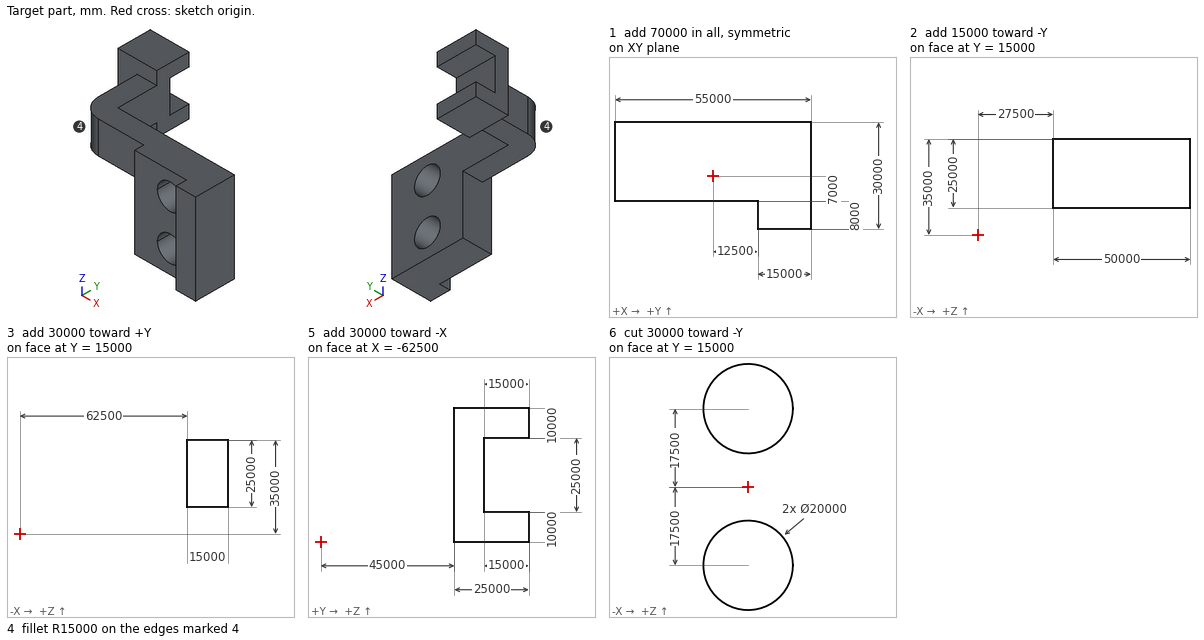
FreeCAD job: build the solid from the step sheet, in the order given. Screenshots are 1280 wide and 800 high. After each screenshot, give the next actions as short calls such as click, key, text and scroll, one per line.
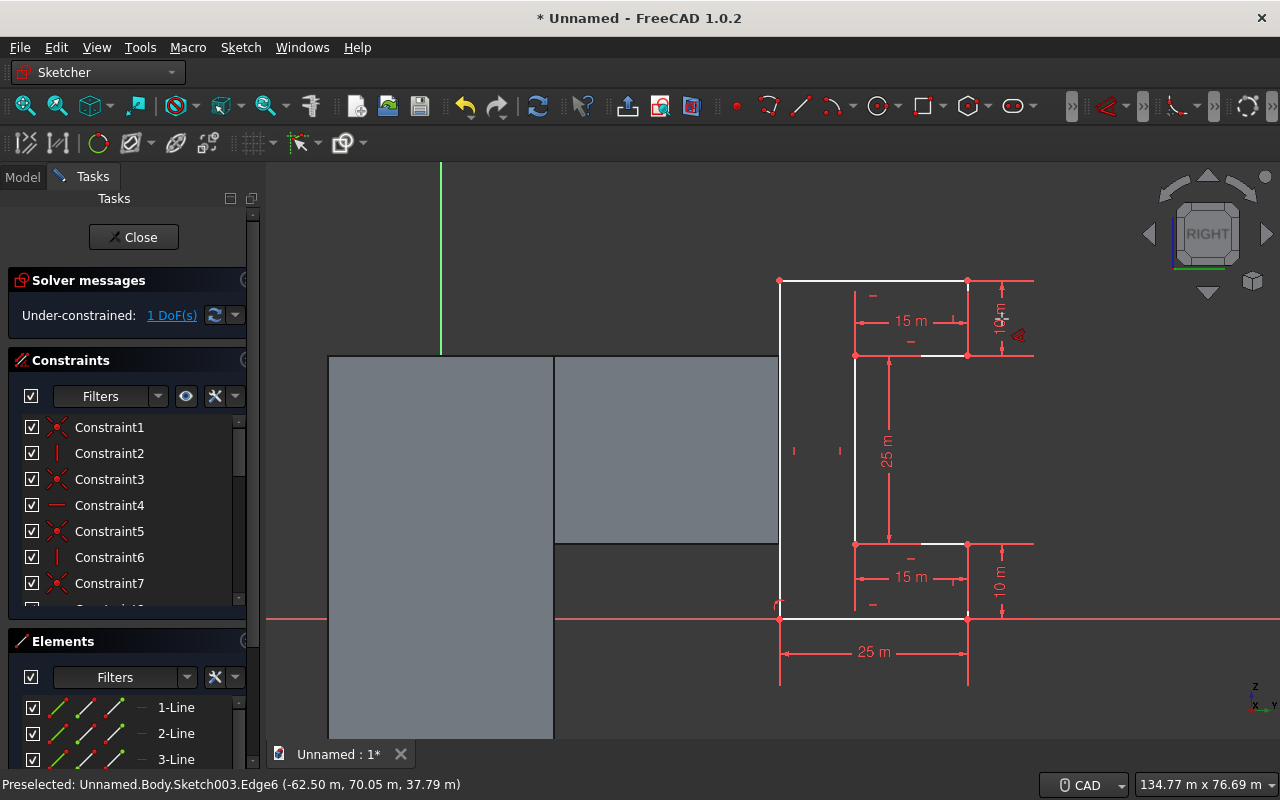
click(780, 619)
click(610, 653)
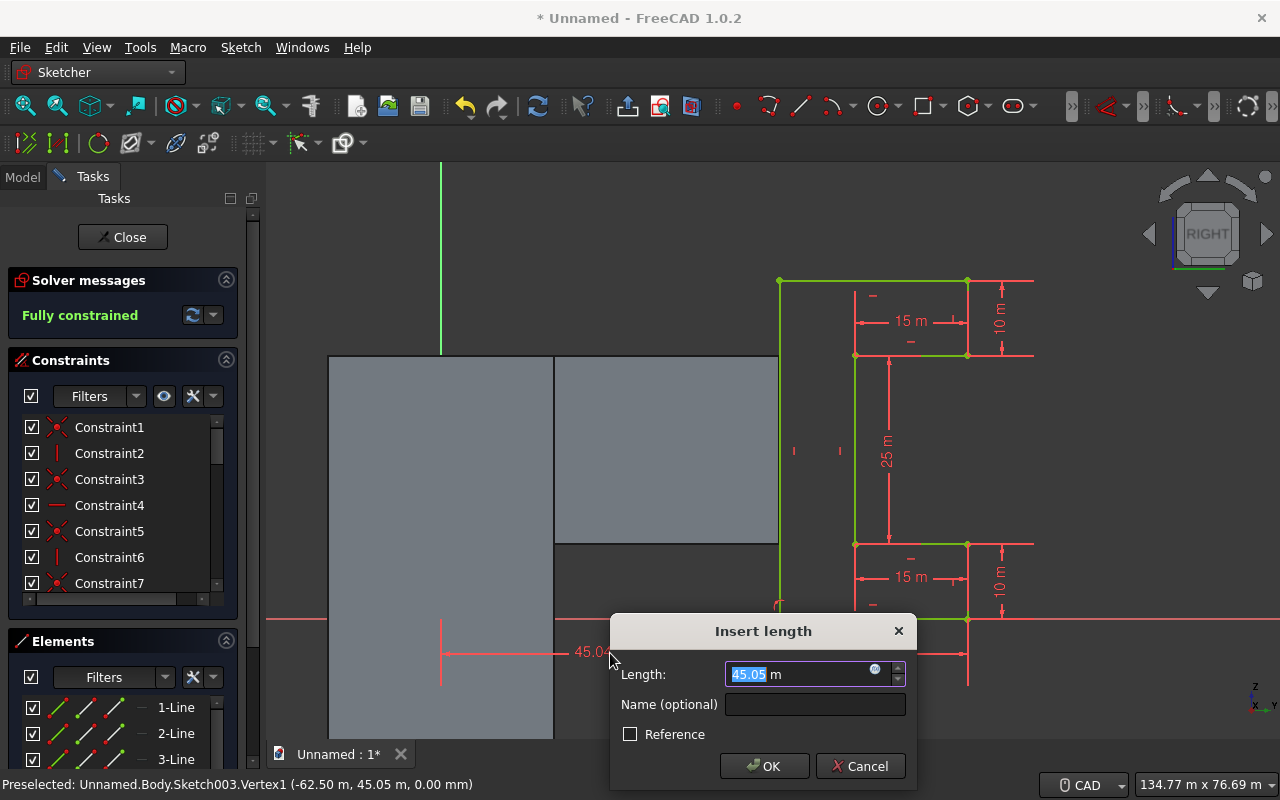
key(ctrl+a)
text(45000 mm)
key(Return)
key(Escape)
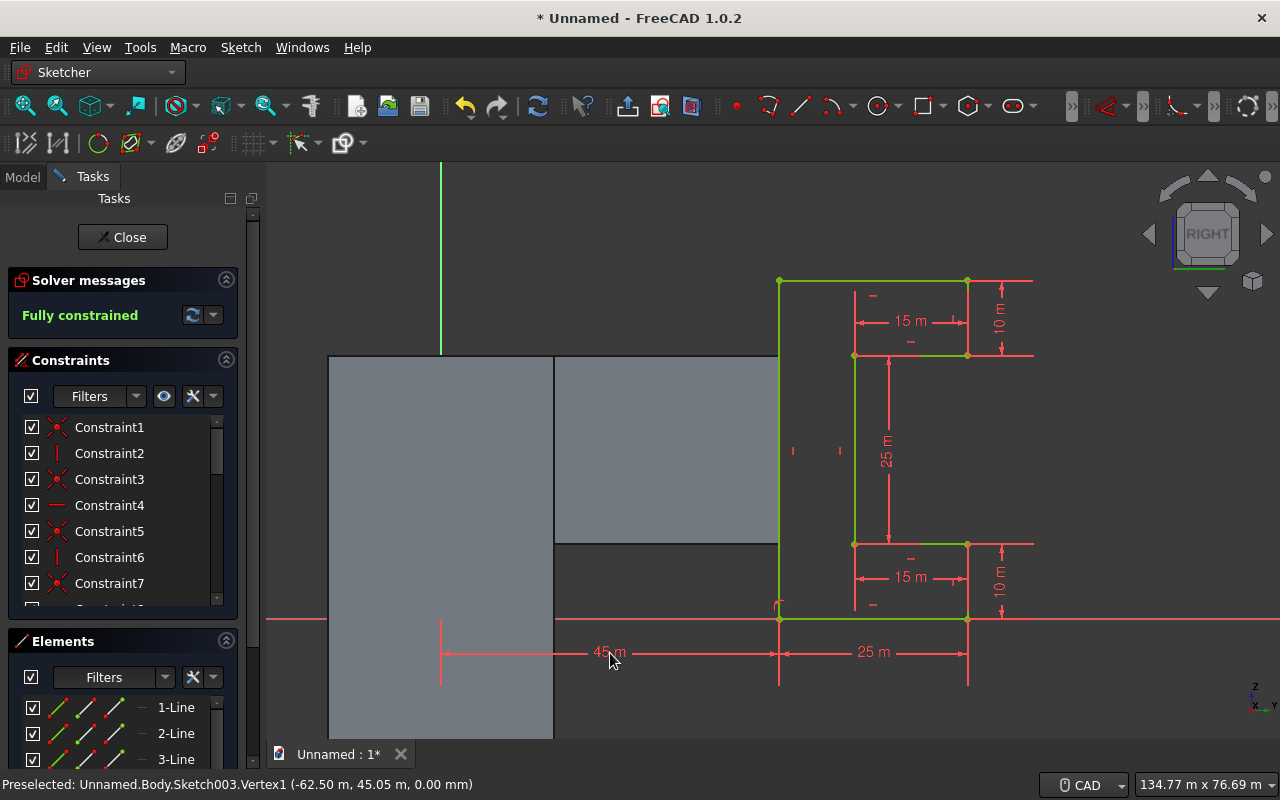
click(123, 237)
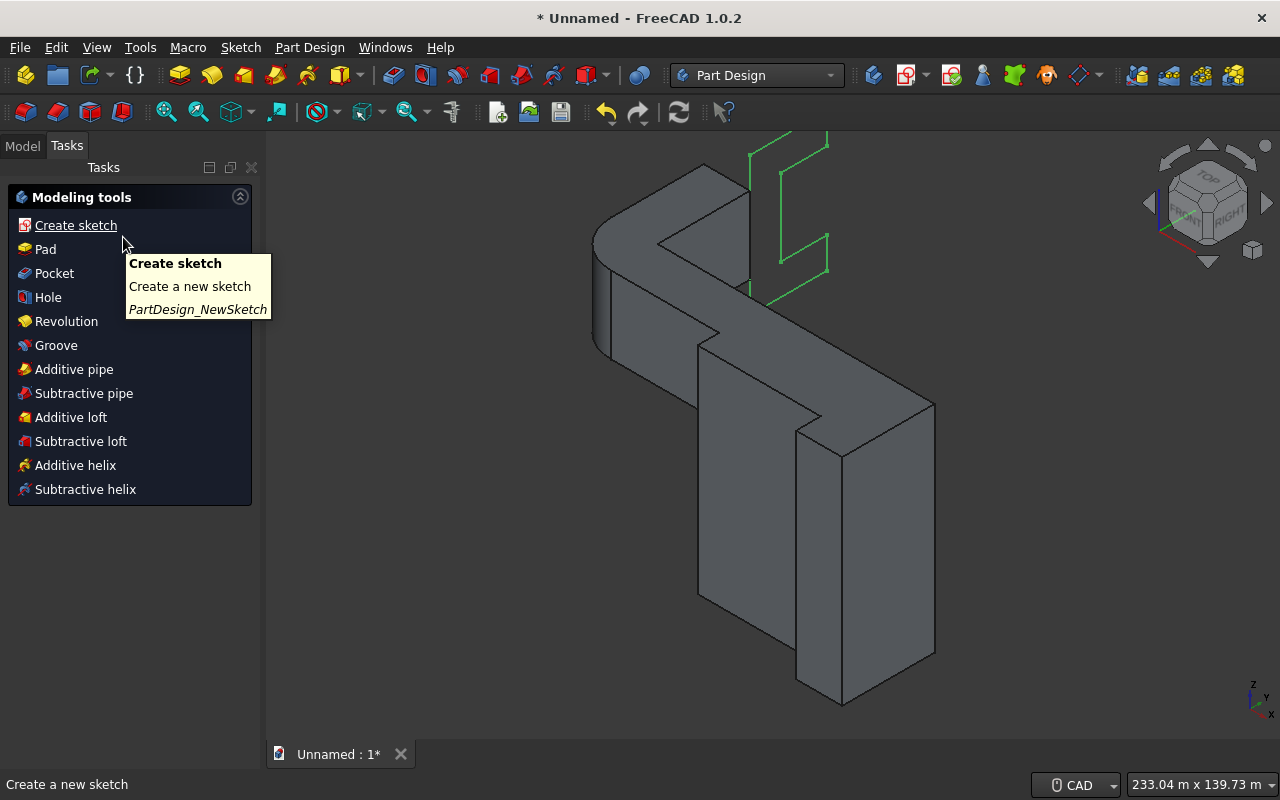
click(180, 76)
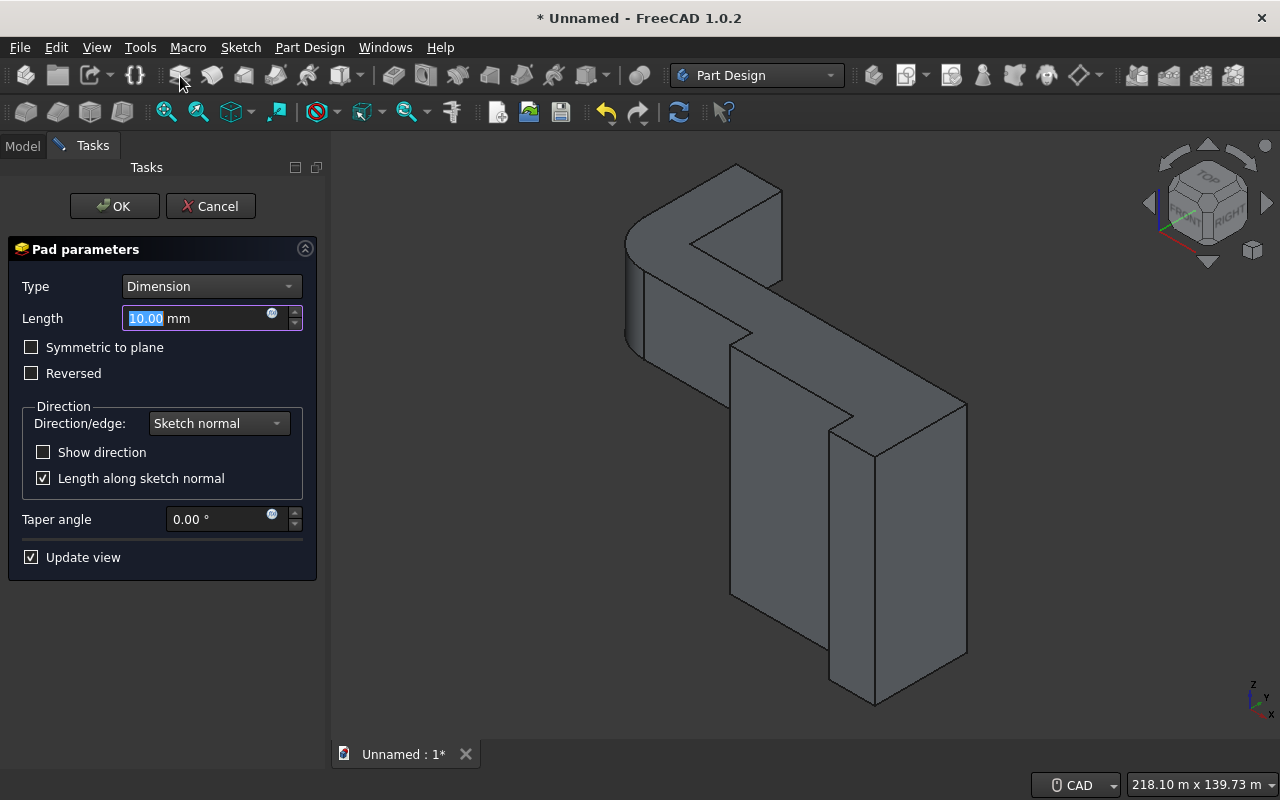
text(30000)
key(Tab)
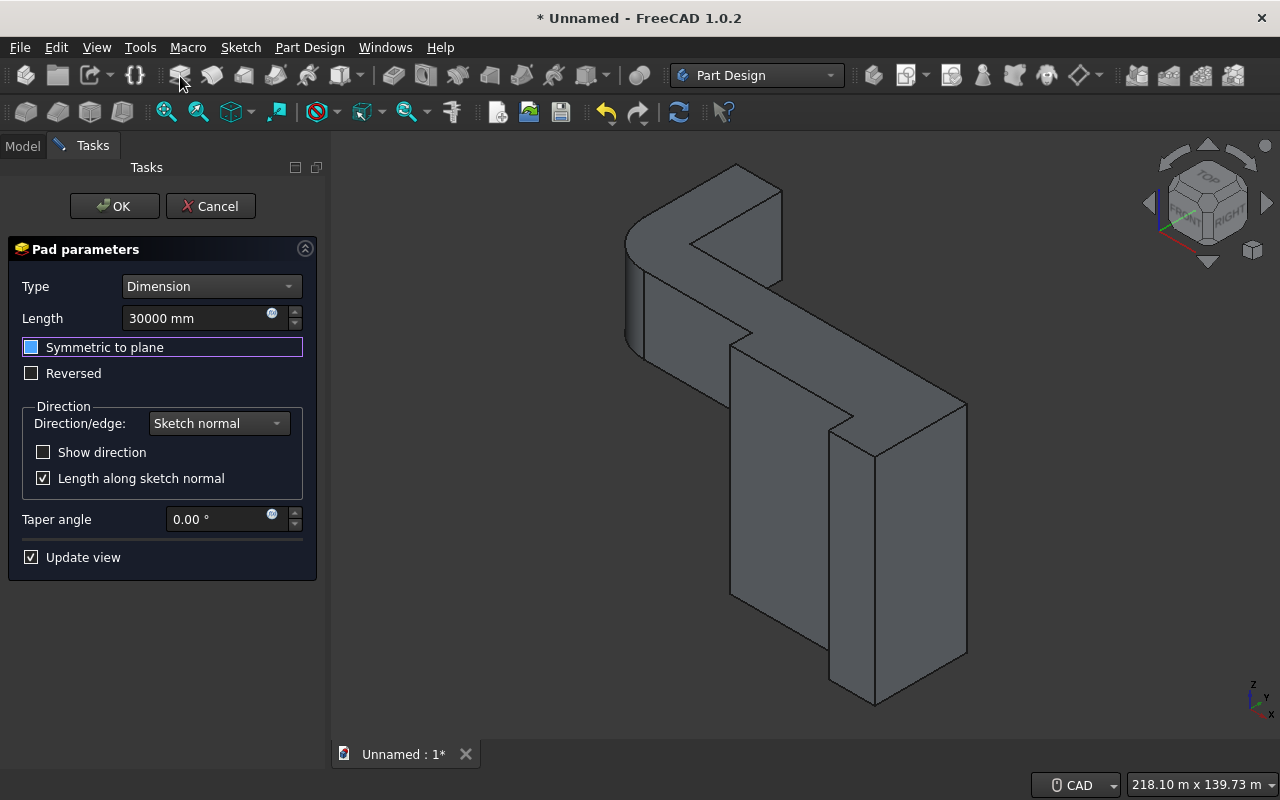
click(30, 373)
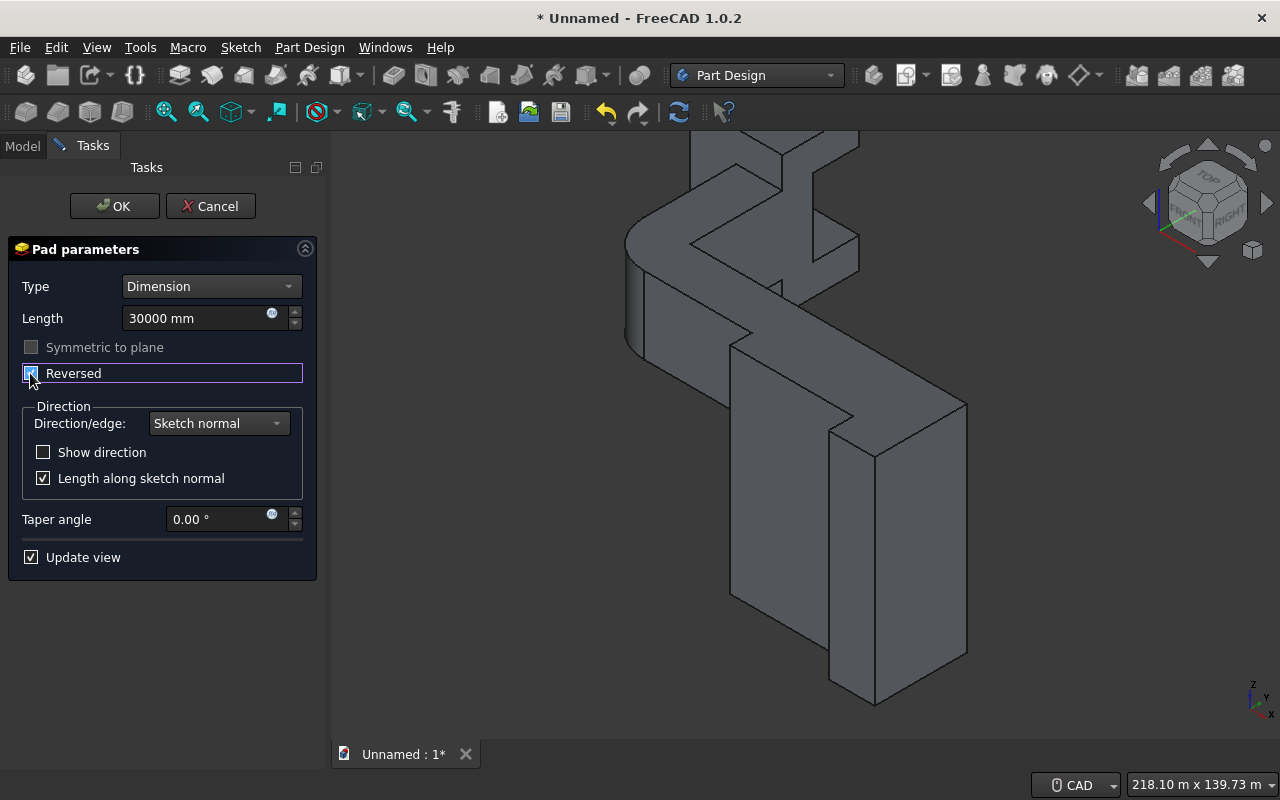
click(115, 206)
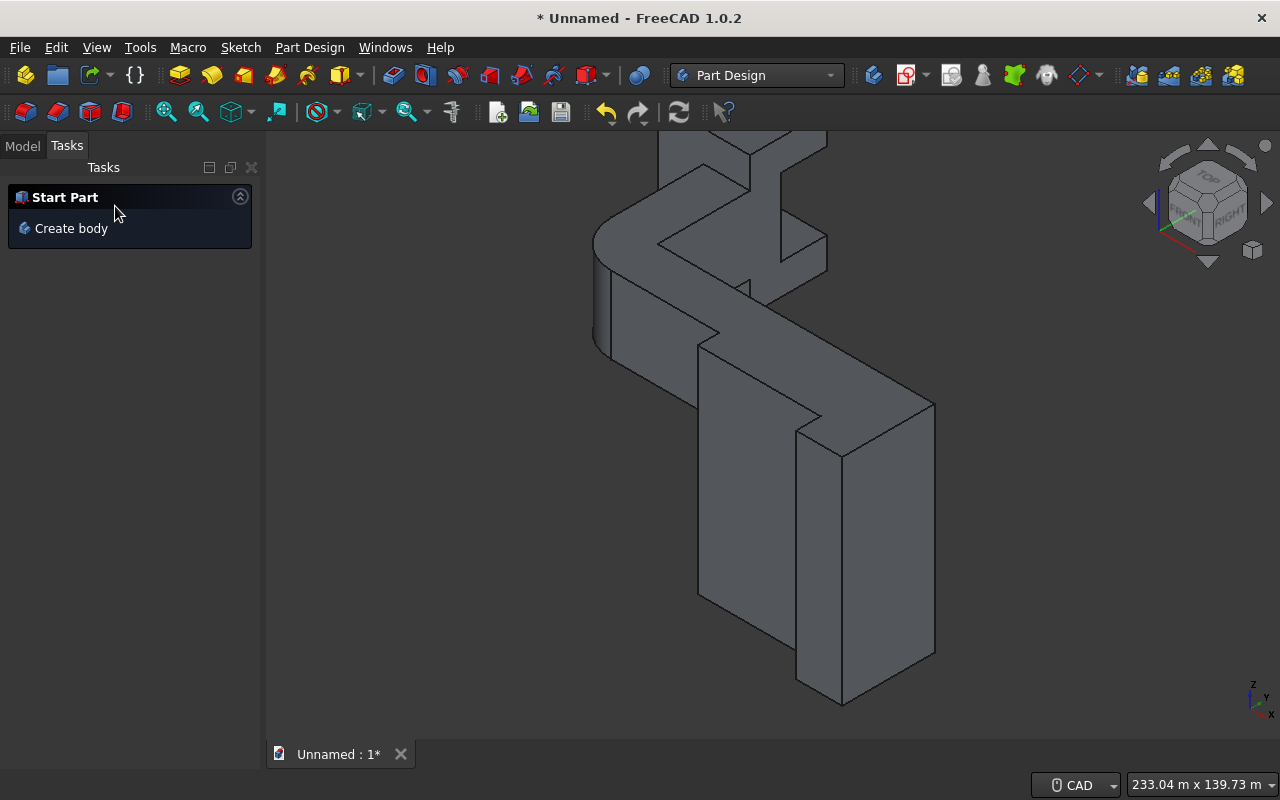
key(v)
key(f)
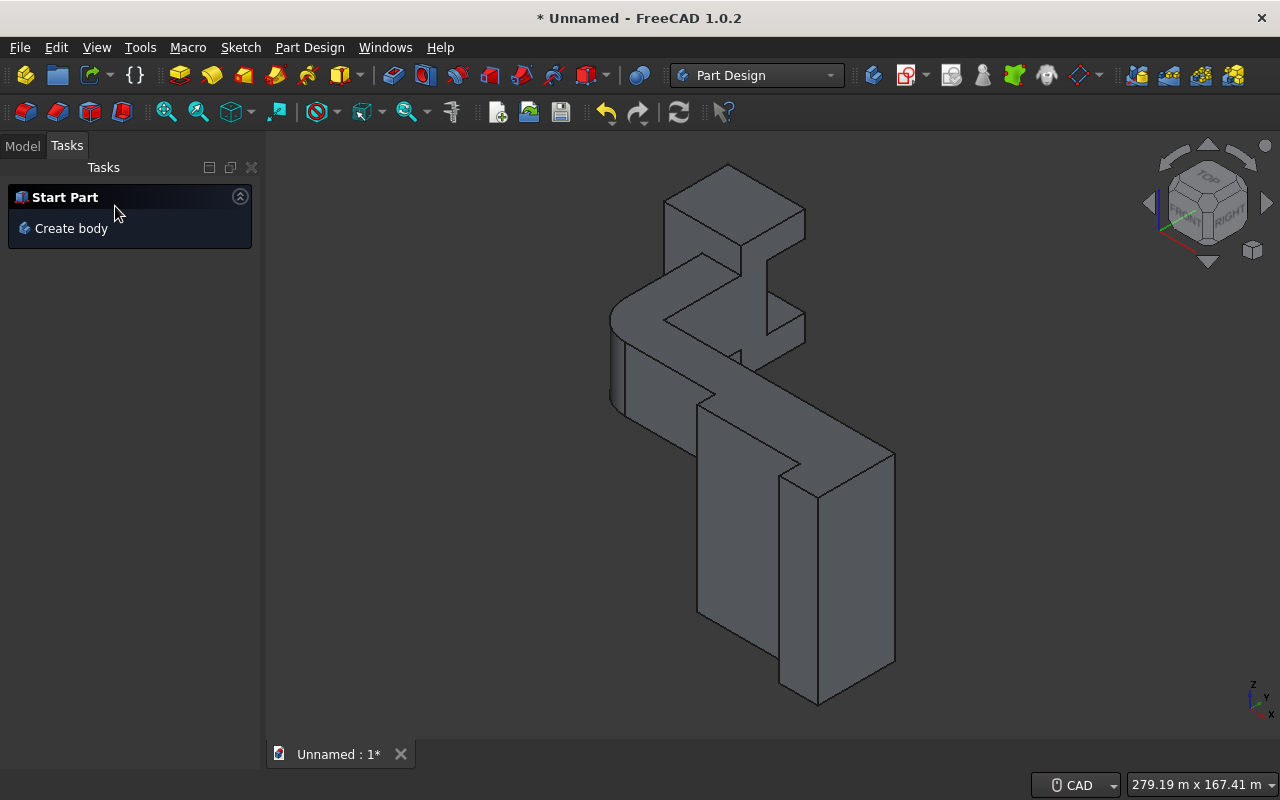
key(4)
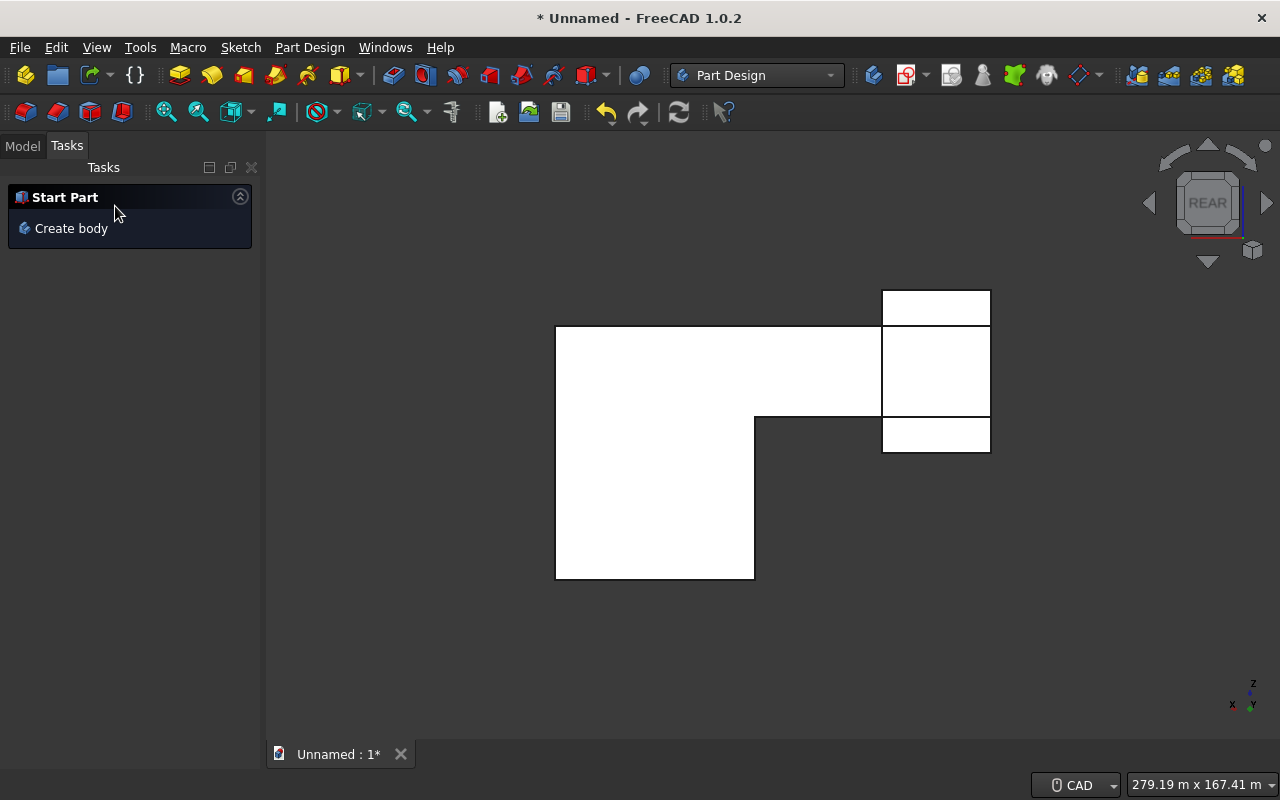
click(672, 416)